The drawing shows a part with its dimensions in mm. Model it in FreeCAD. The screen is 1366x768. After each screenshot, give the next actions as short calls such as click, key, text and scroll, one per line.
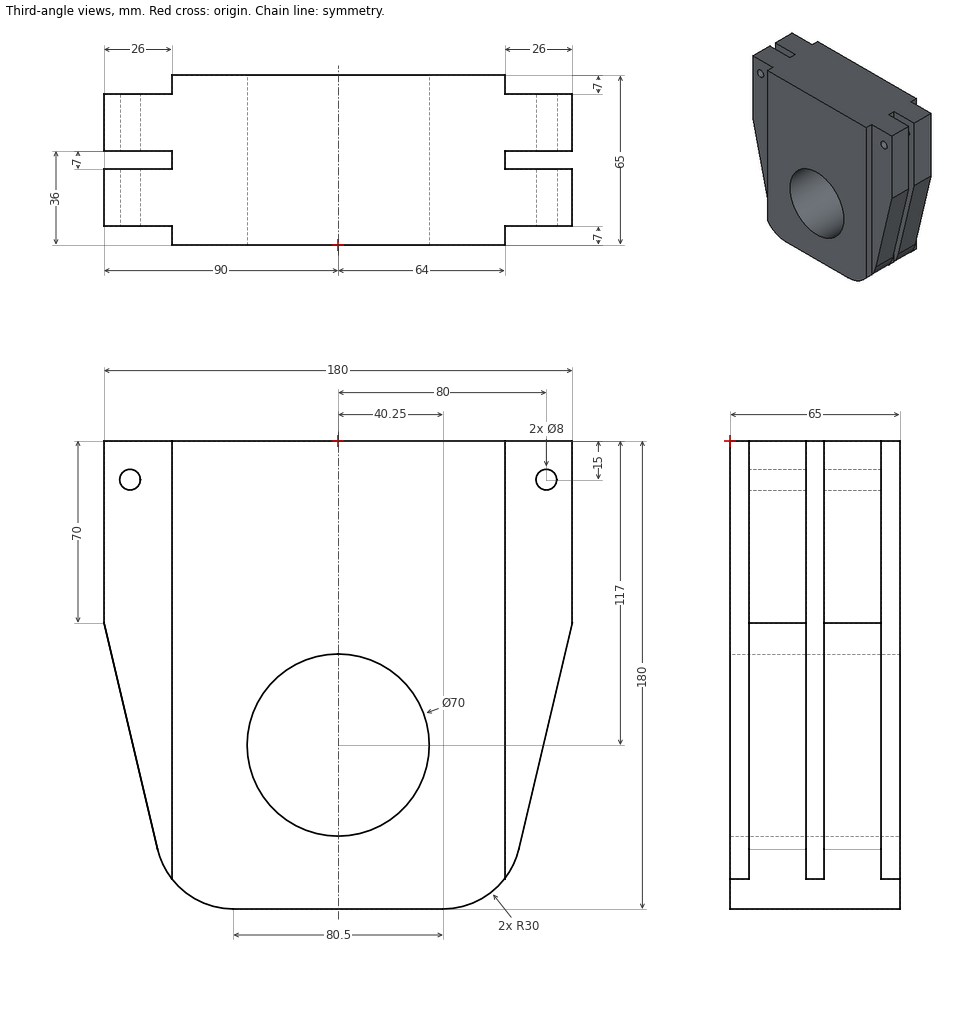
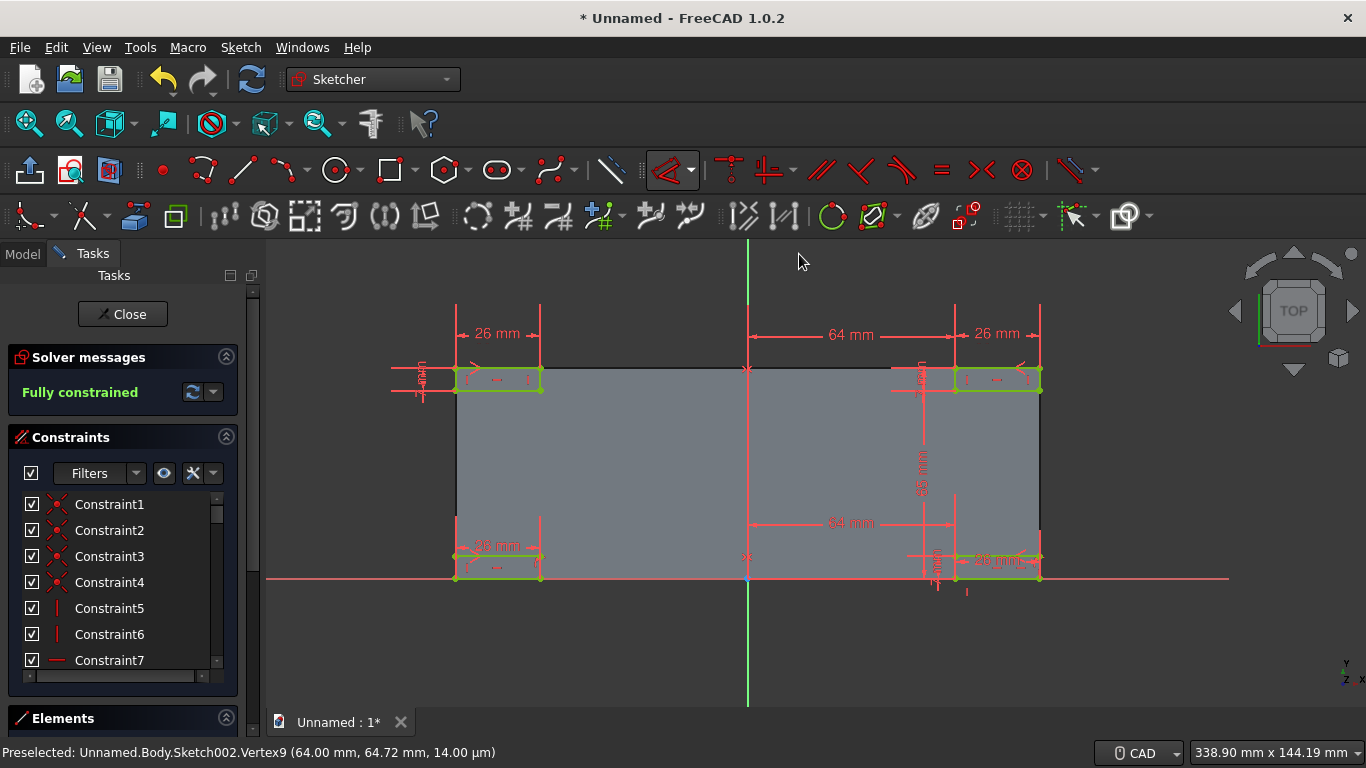
click(123, 314)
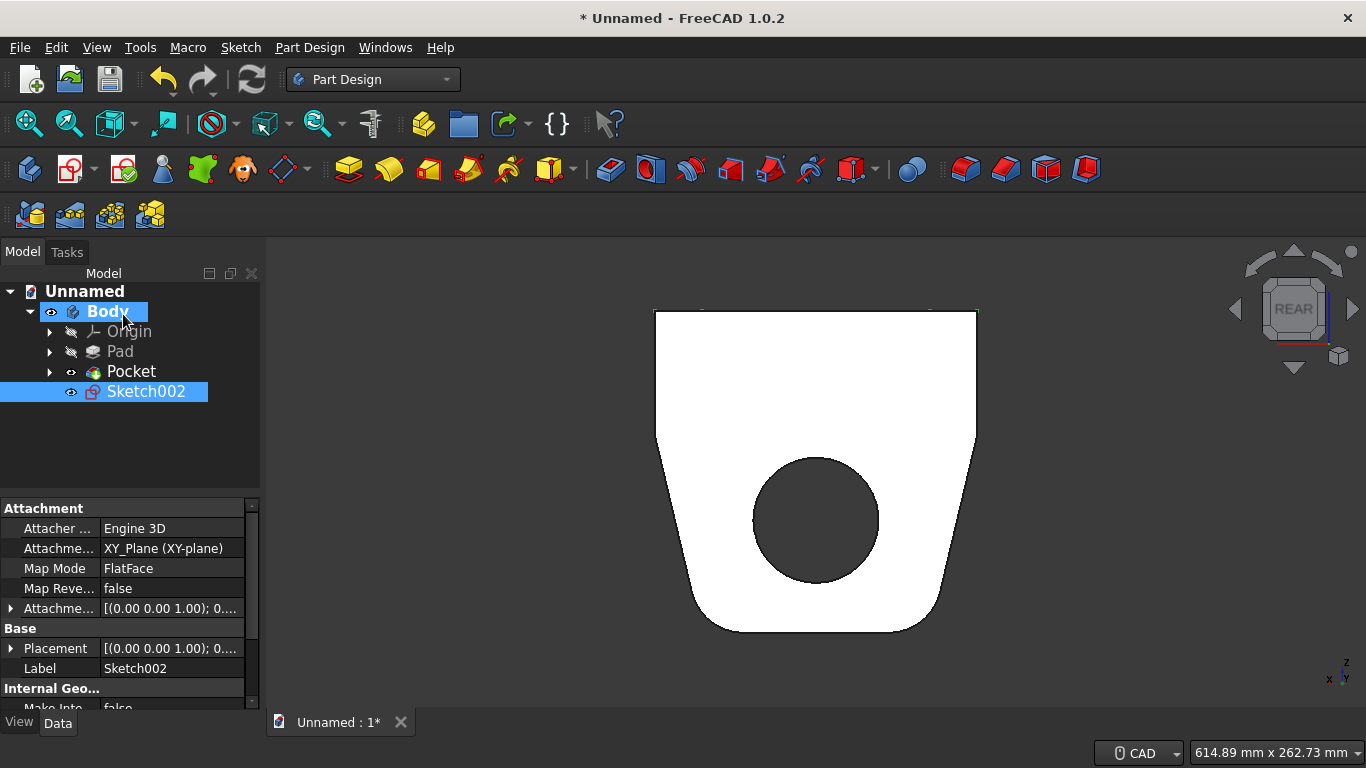
click(612, 170)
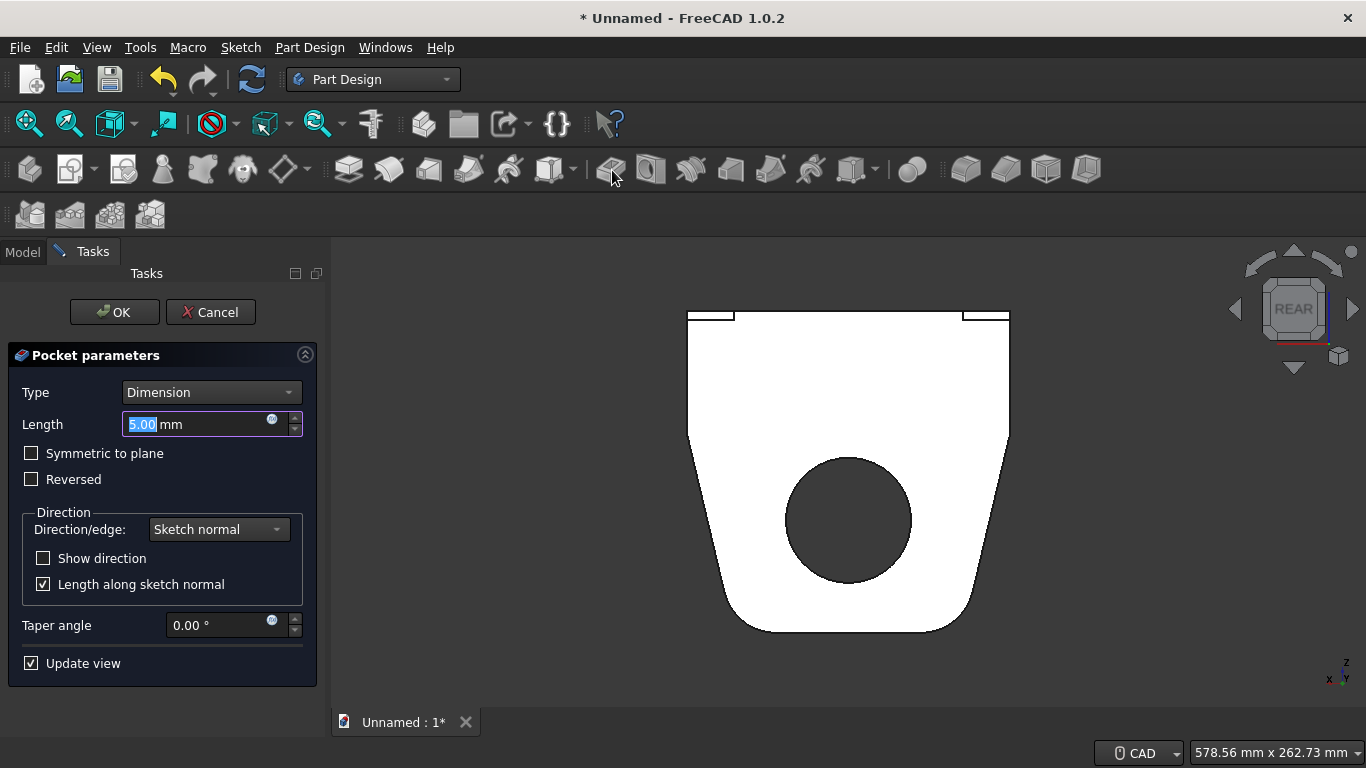
click(212, 392)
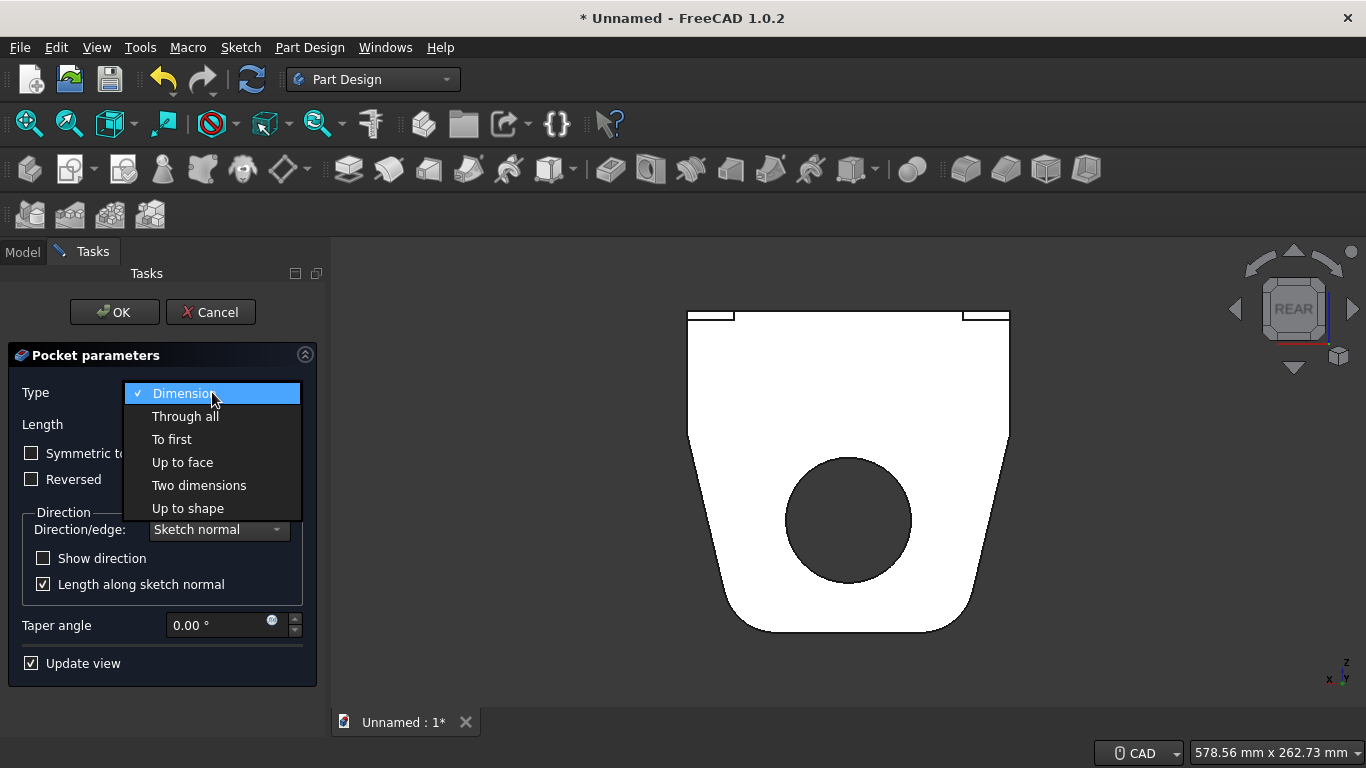
click(212, 416)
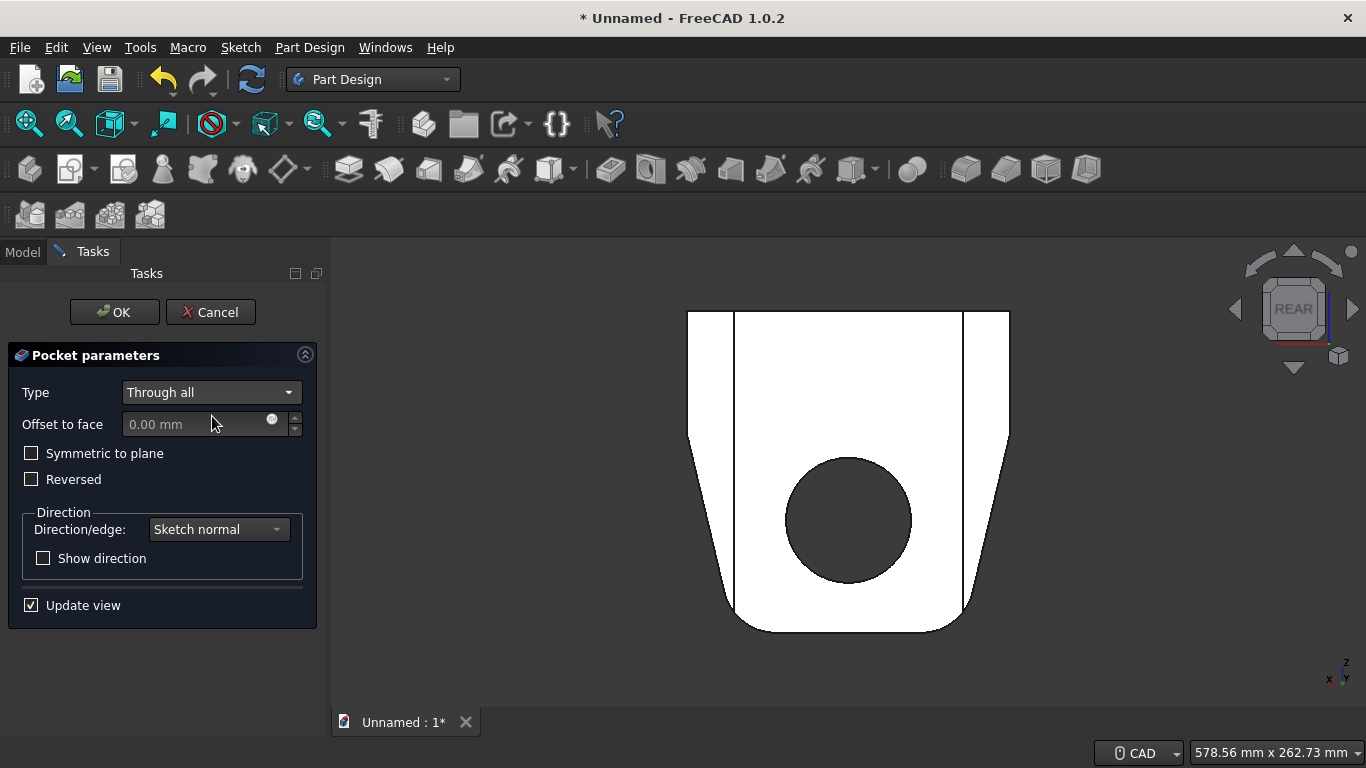
click(115, 312)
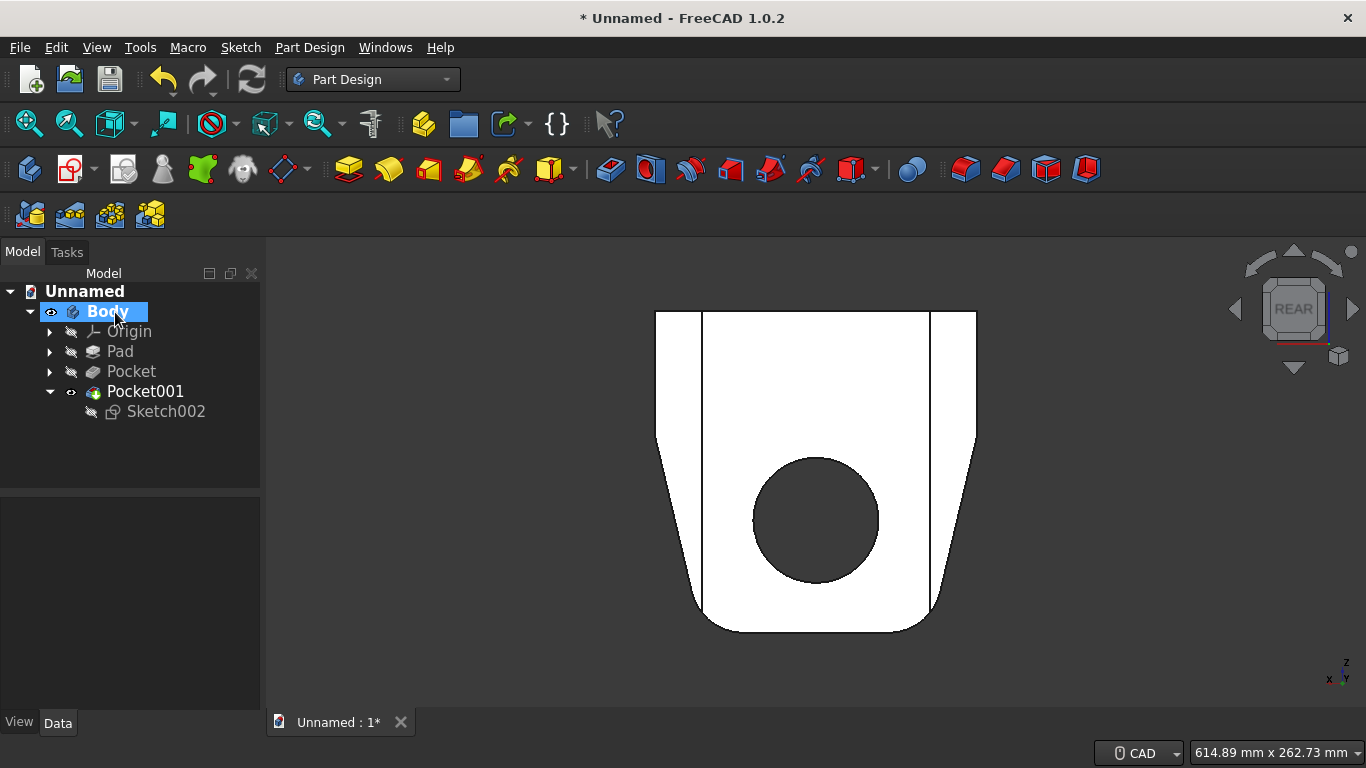
key(0)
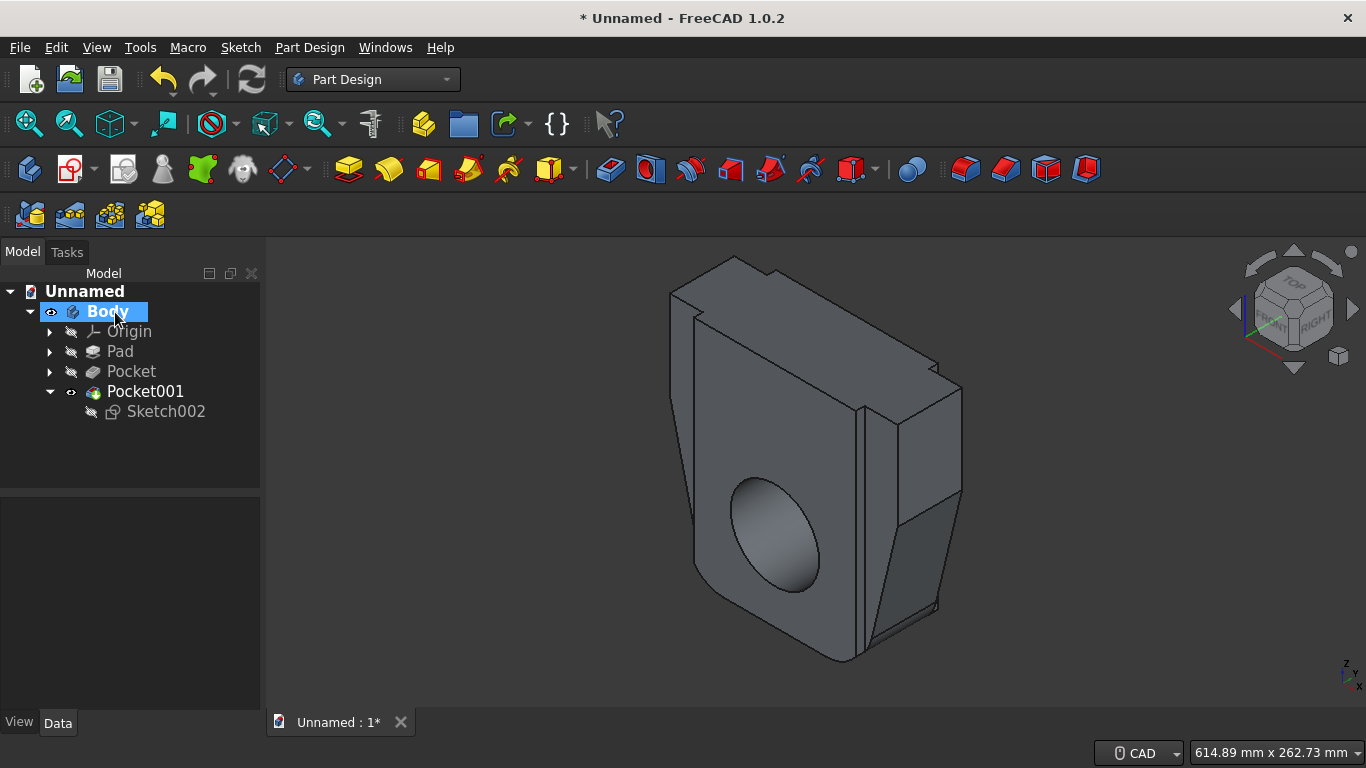
key(1)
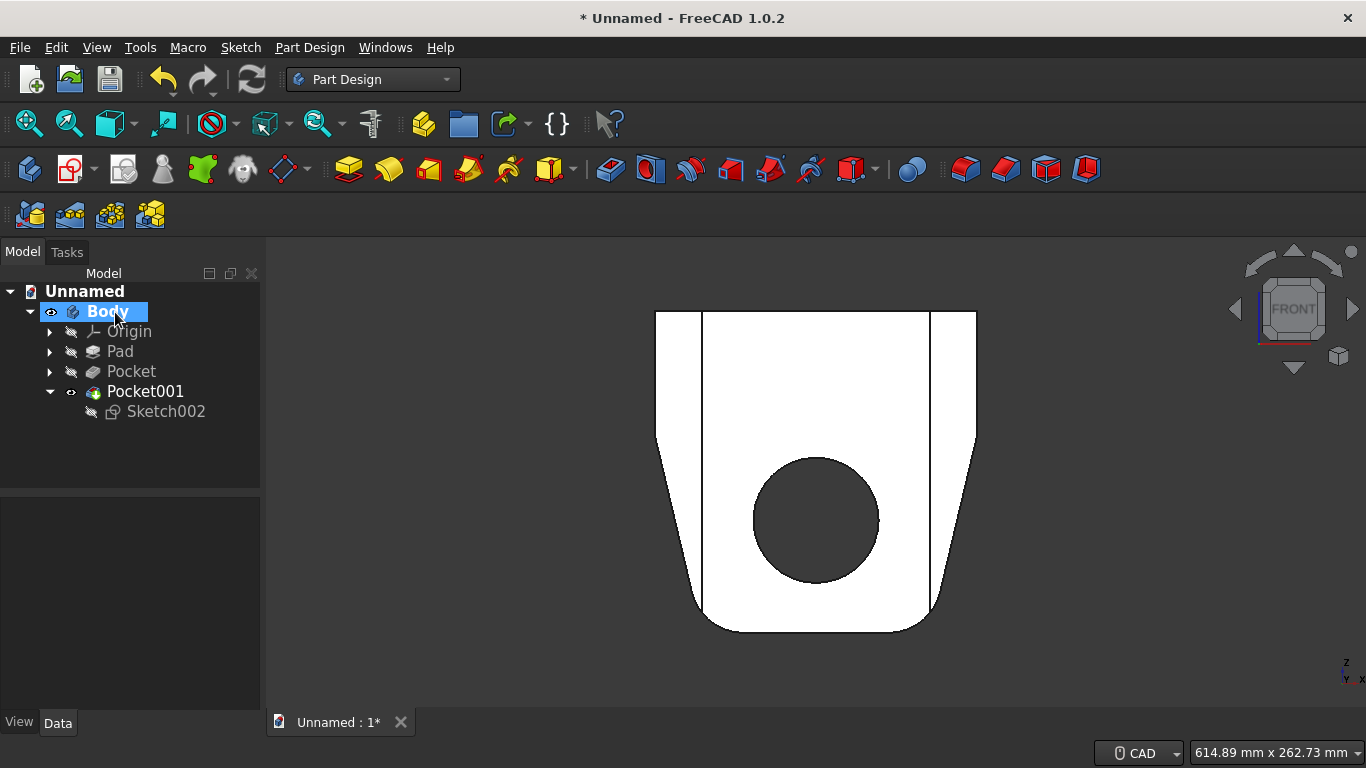
click(678, 375)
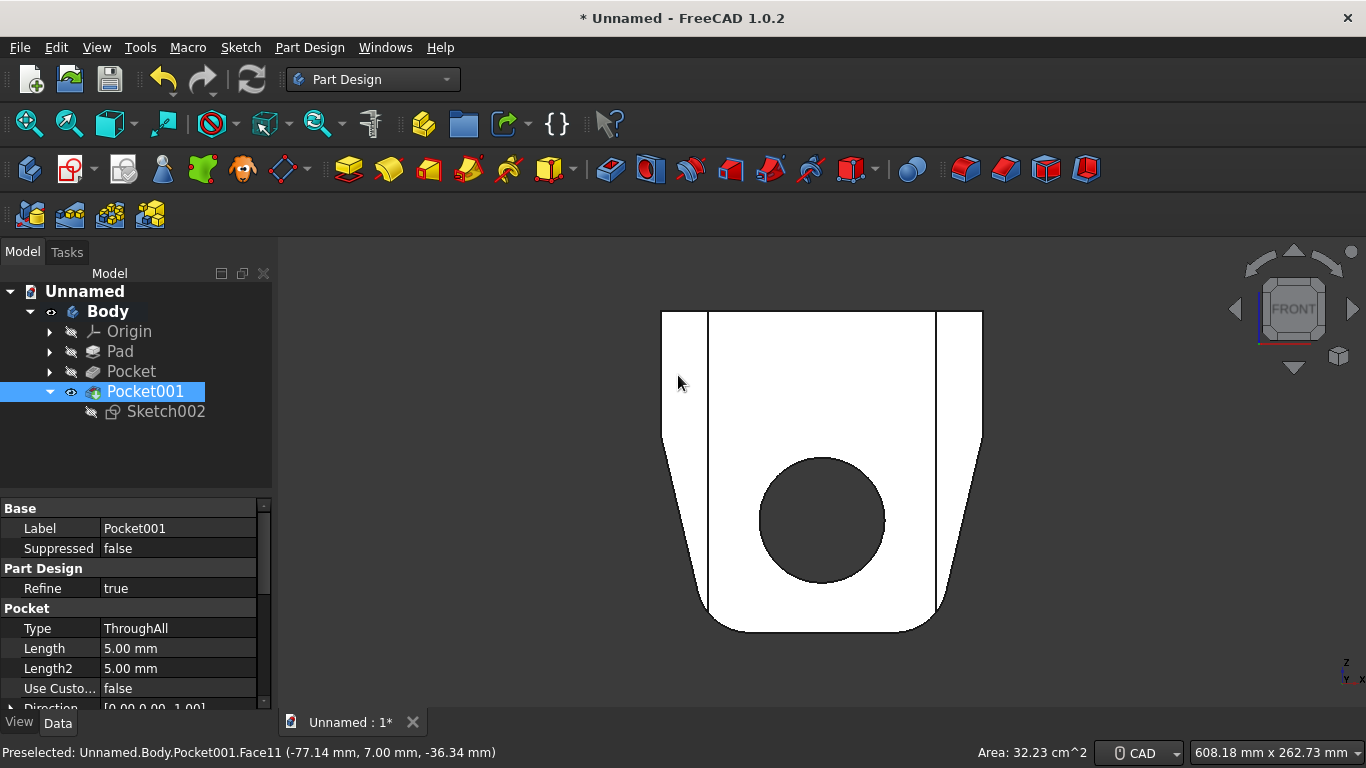
click(70, 170)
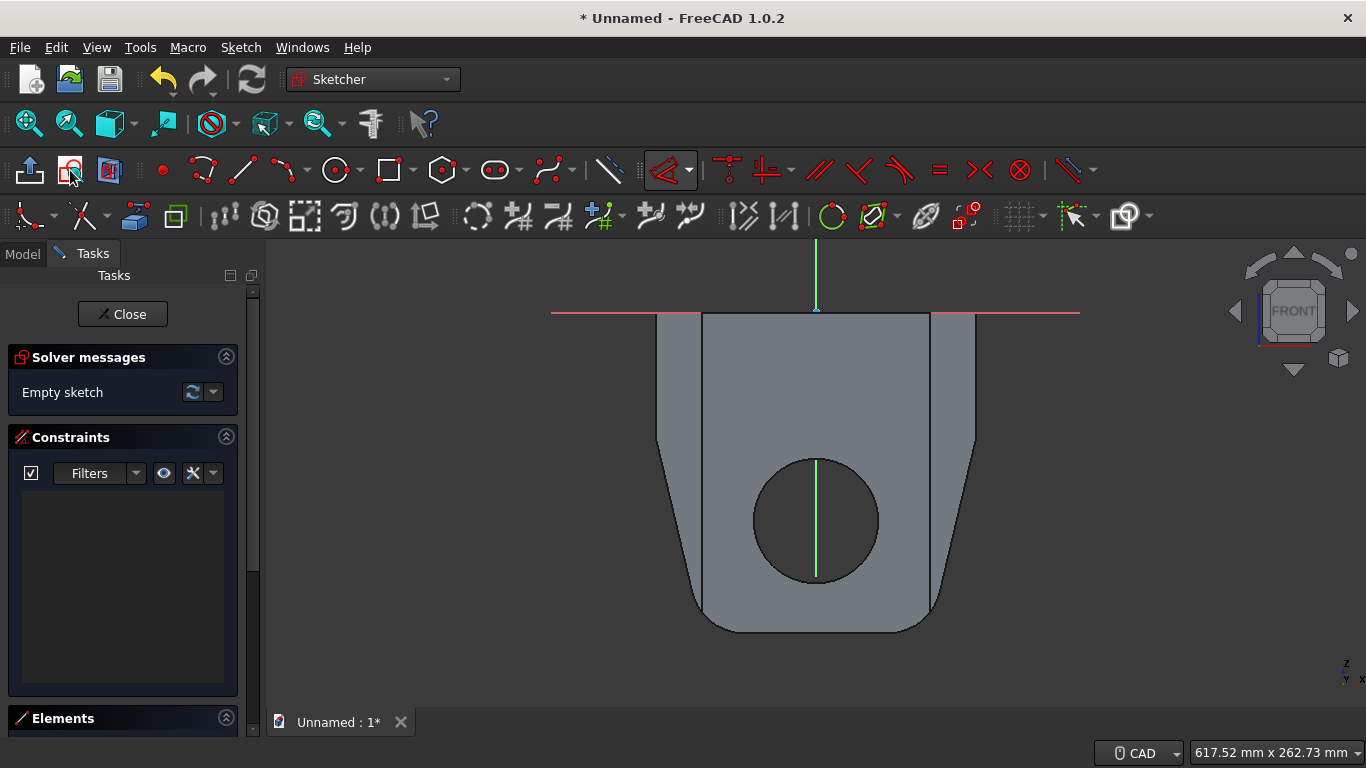
click(110, 170)